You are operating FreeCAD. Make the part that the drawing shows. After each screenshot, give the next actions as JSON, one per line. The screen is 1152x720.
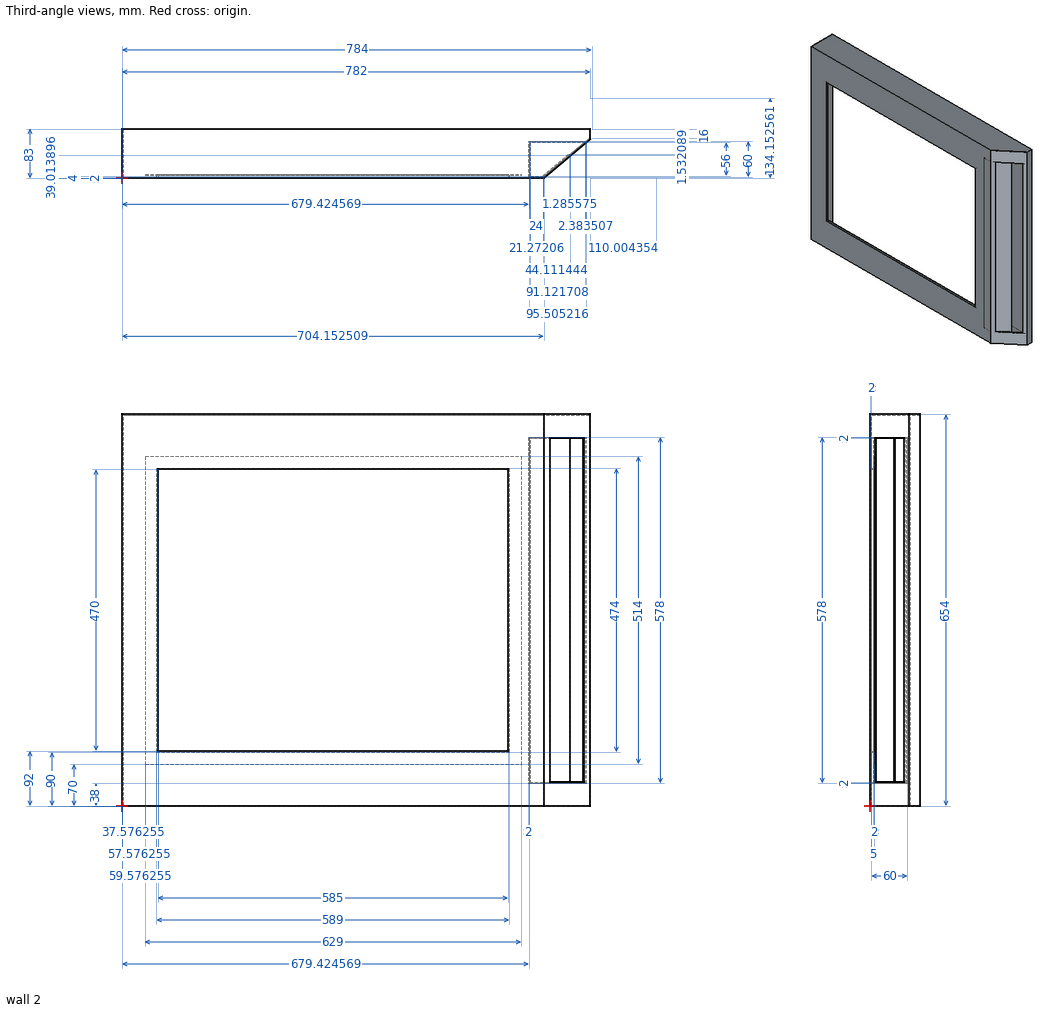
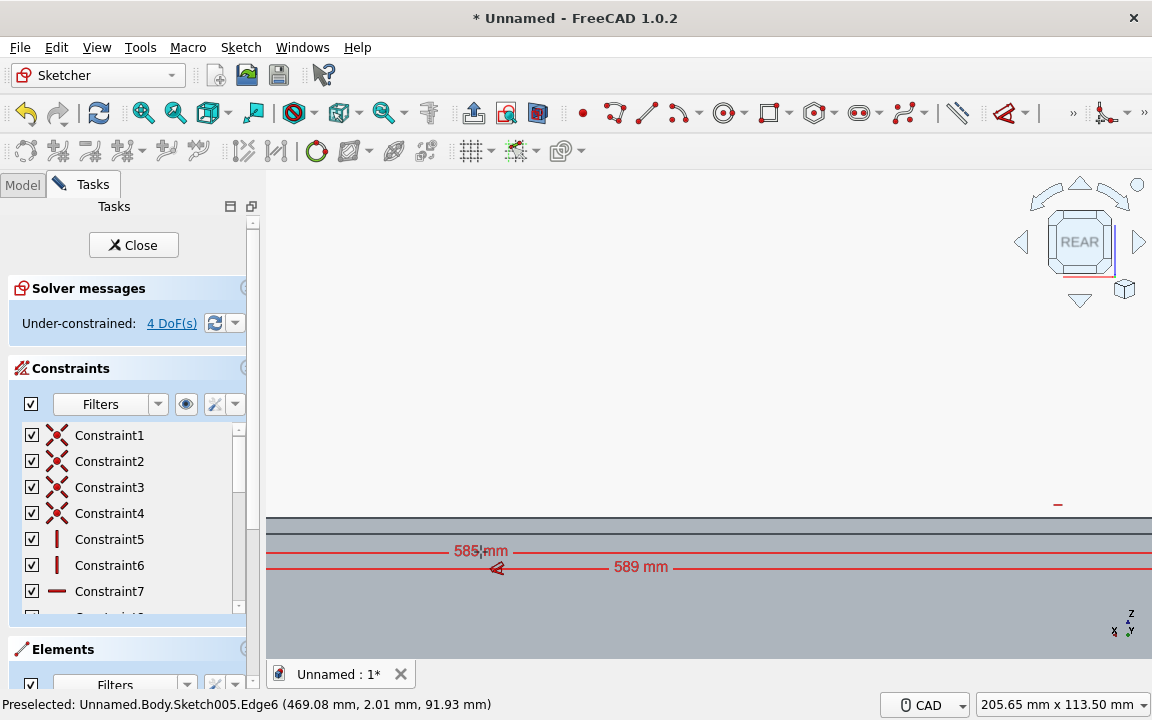
{"action": "scroll", "coordinate": [555, 526], "scroll_direction": "down", "scroll_amount": 10}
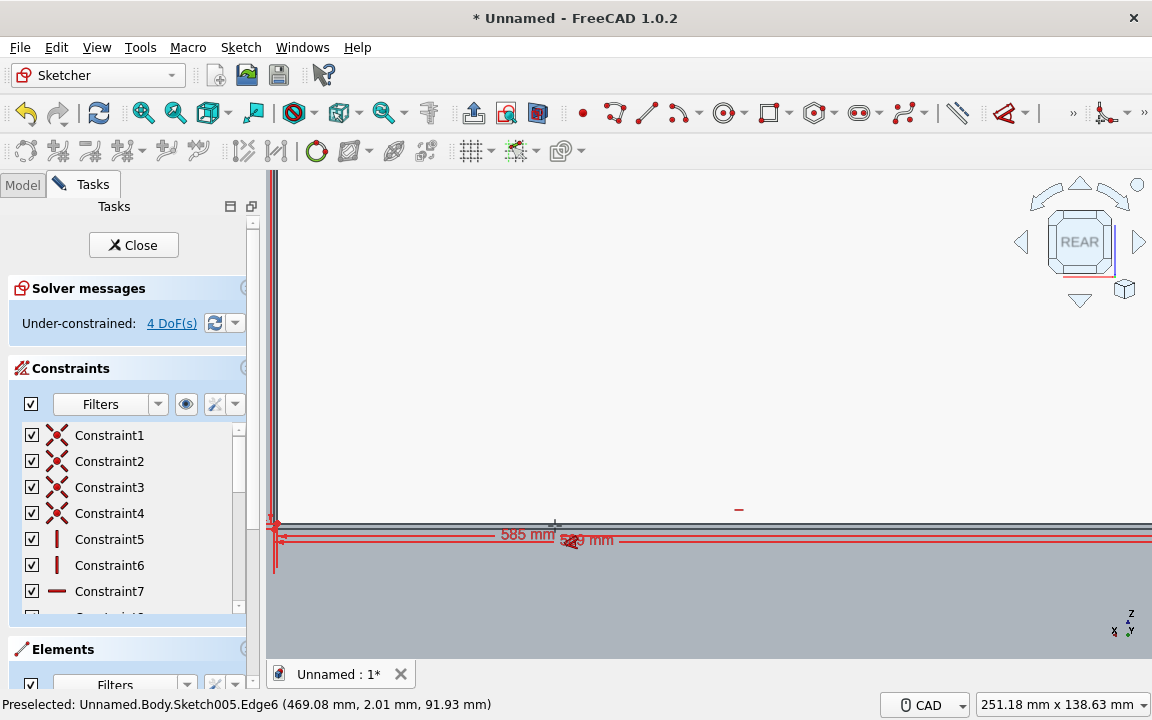
{"action": "scroll", "coordinate": [452, 528], "scroll_direction": "up", "scroll_amount": 9}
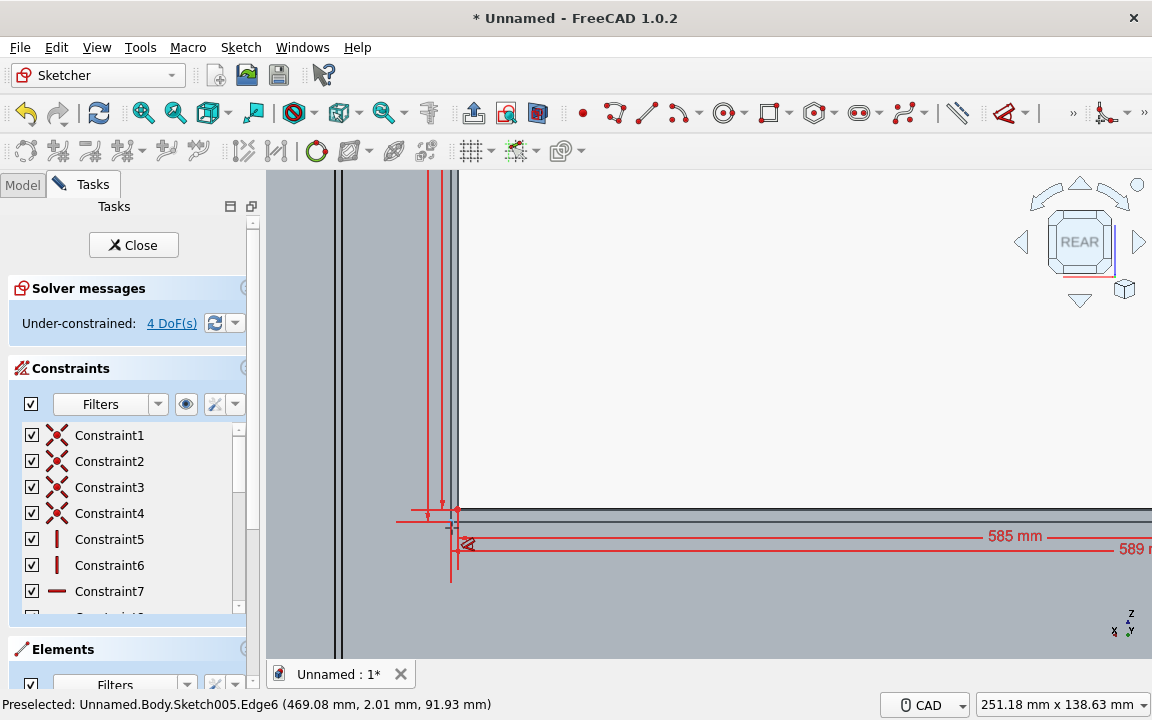
{"action": "left_click", "coordinate": [451, 522]}
{"action": "left_click", "coordinate": [417, 577]}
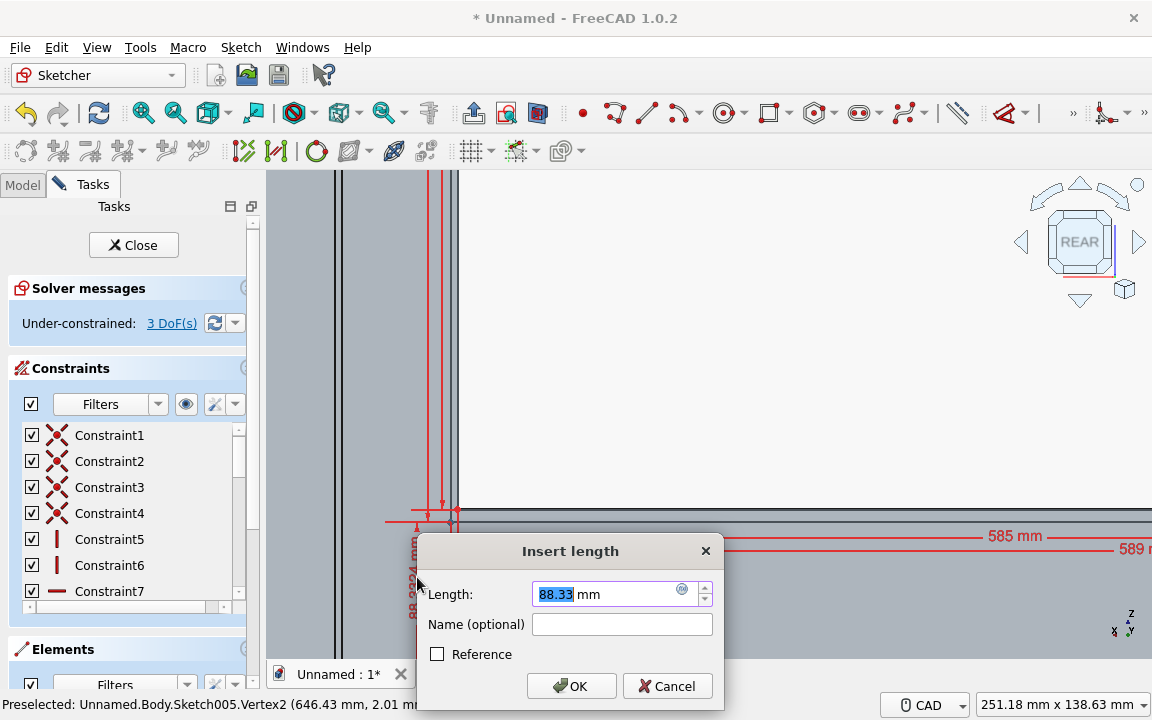
{"action": "type", "text": "90"}
{"action": "key", "text": "Return"}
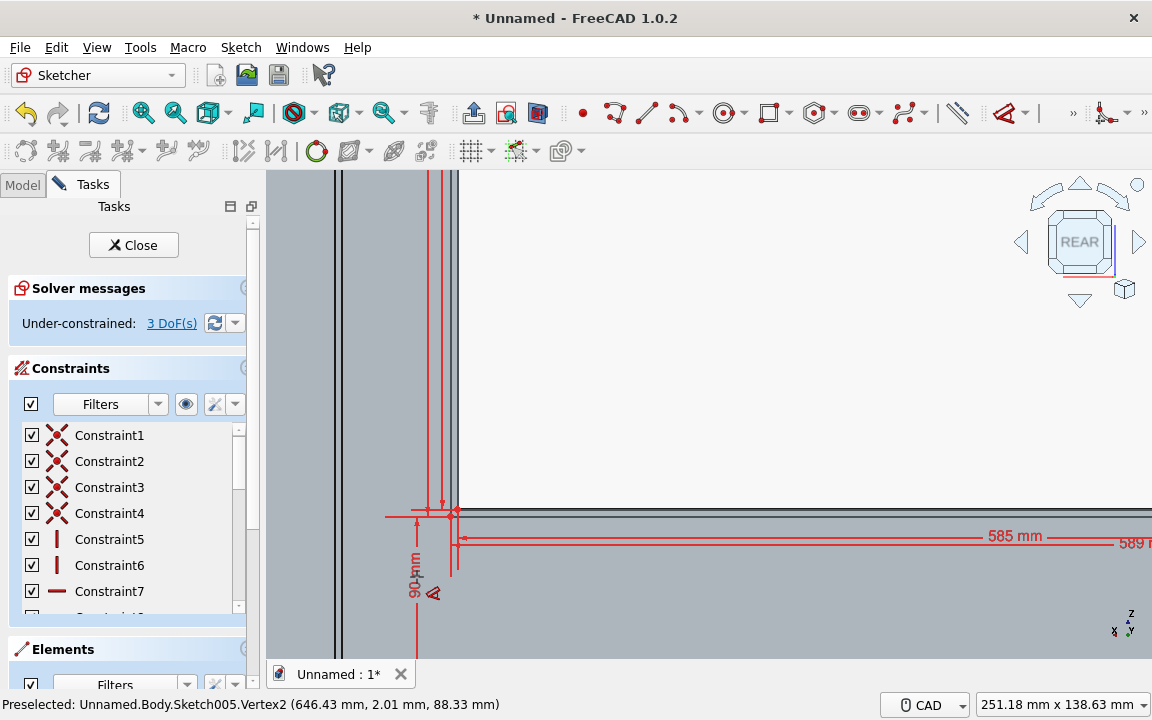
{"action": "scroll", "coordinate": [458, 510], "scroll_direction": "up", "scroll_amount": 2}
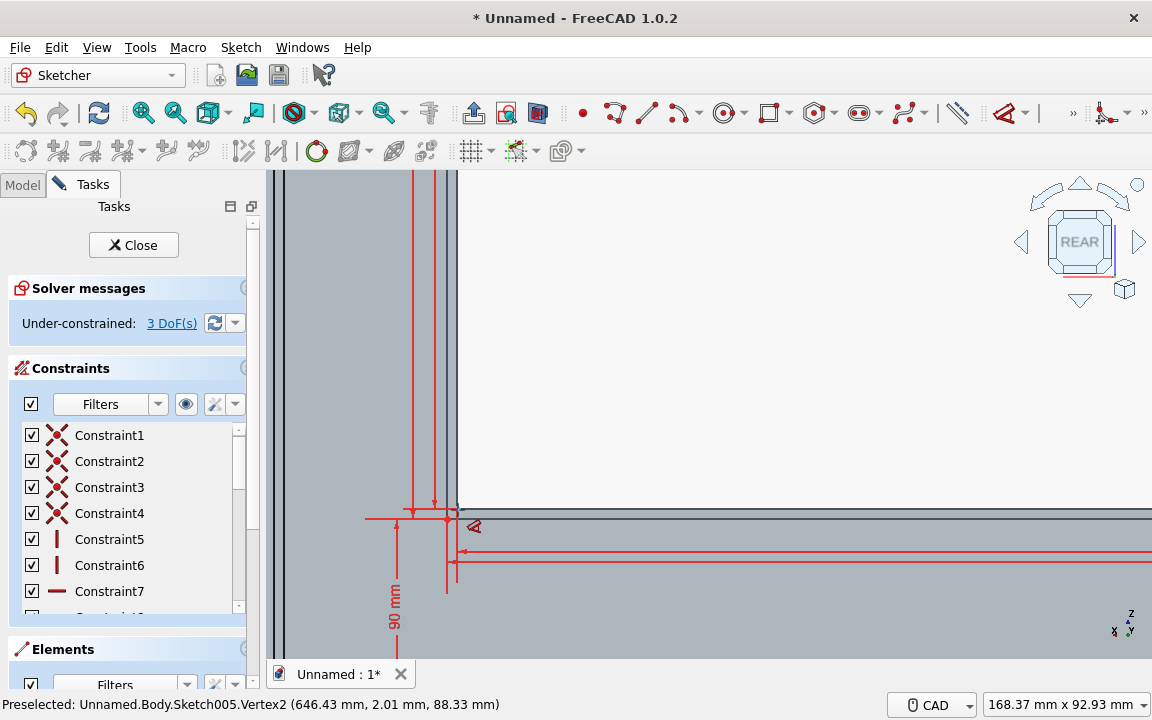
{"action": "left_click", "coordinate": [457, 509]}
{"action": "left_click", "coordinate": [423, 570]}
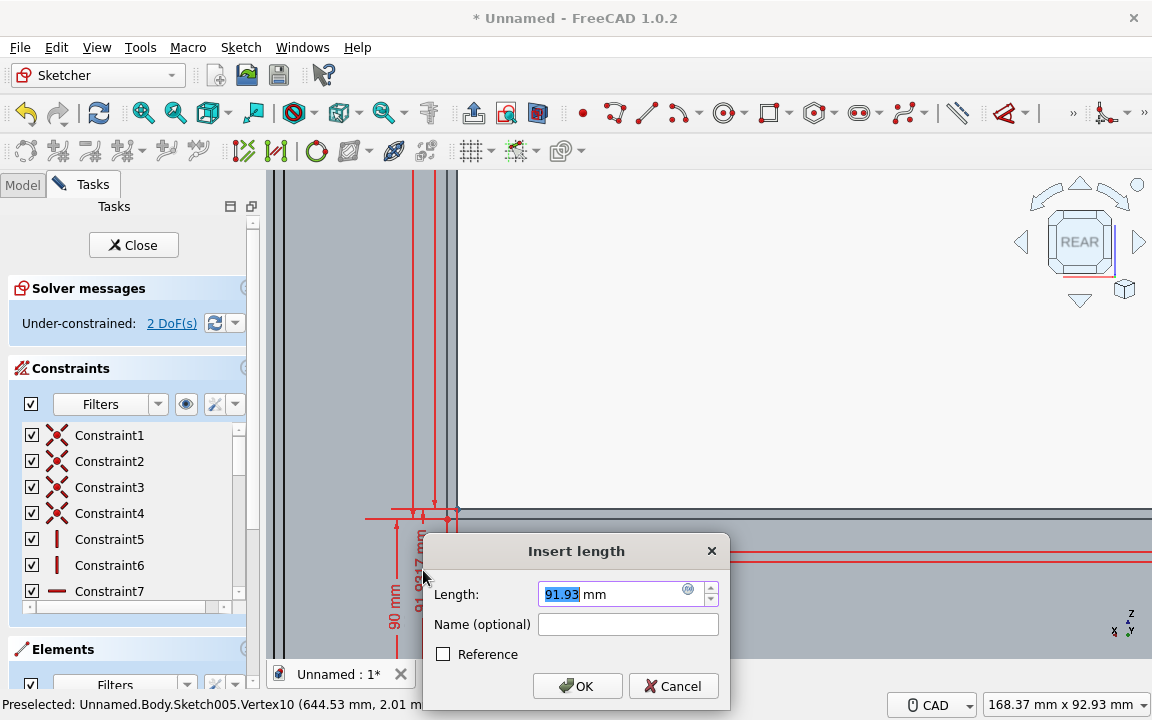
{"action": "type", "text": "92"}
{"action": "key", "text": "Return"}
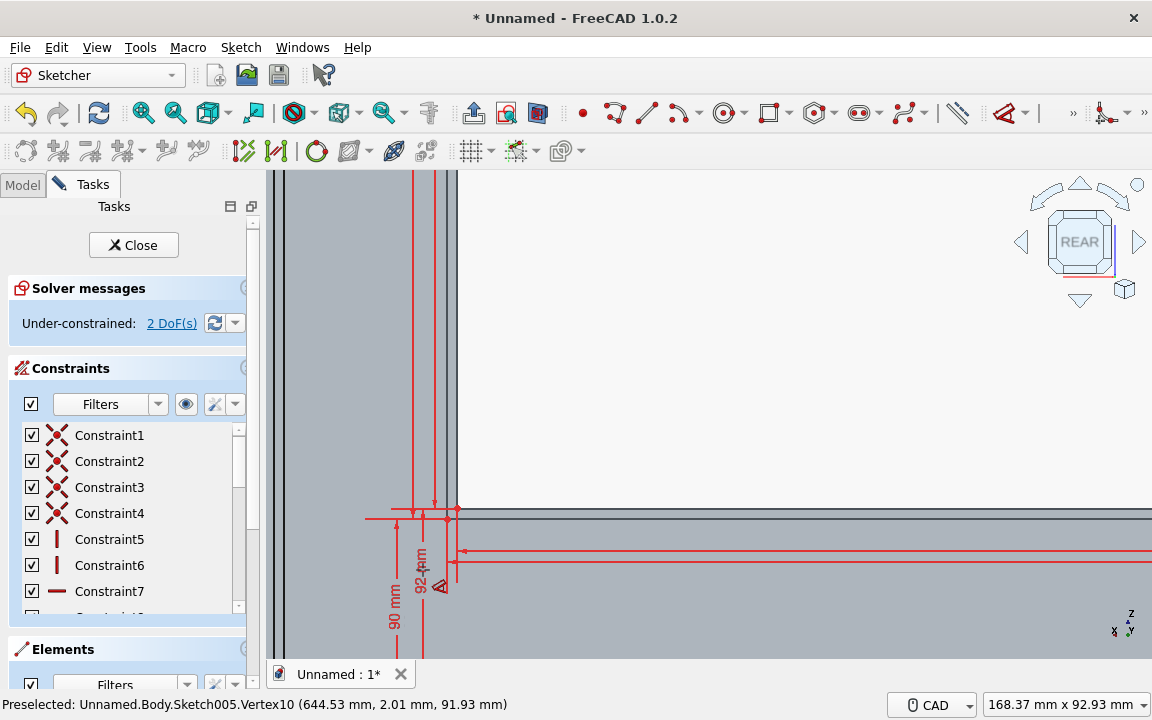
{"action": "scroll", "coordinate": [453, 527], "scroll_direction": "down", "scroll_amount": 11}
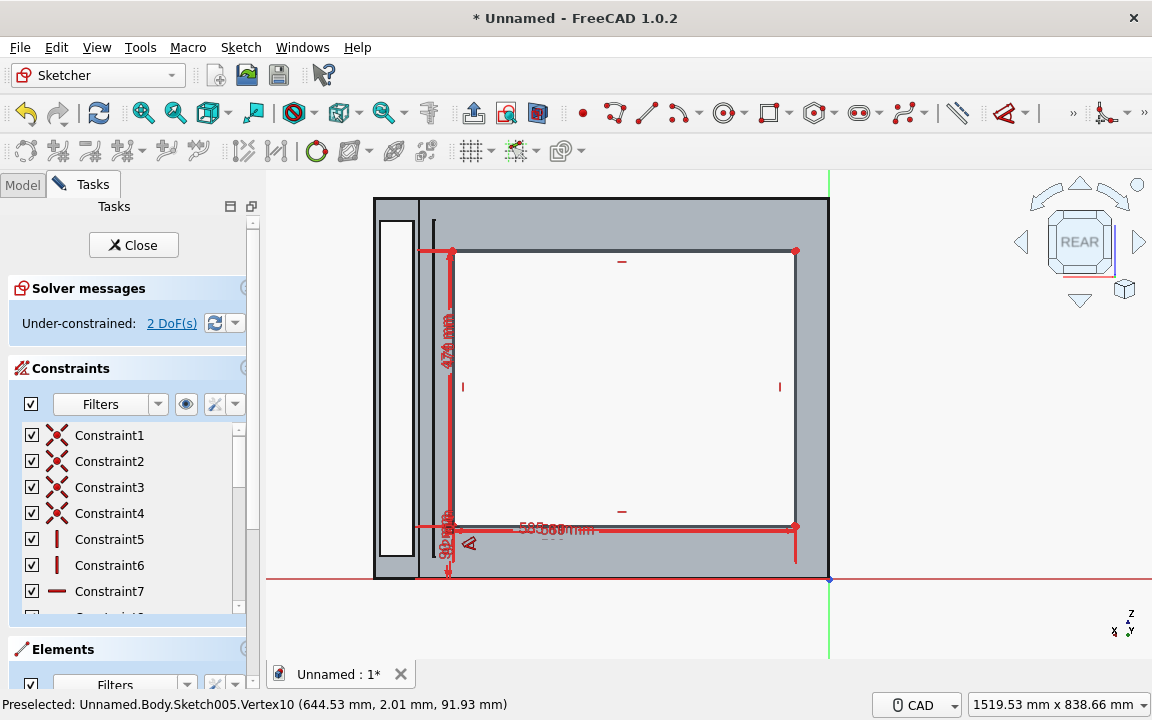
{"action": "scroll", "coordinate": [796, 527], "scroll_direction": "up", "scroll_amount": 10}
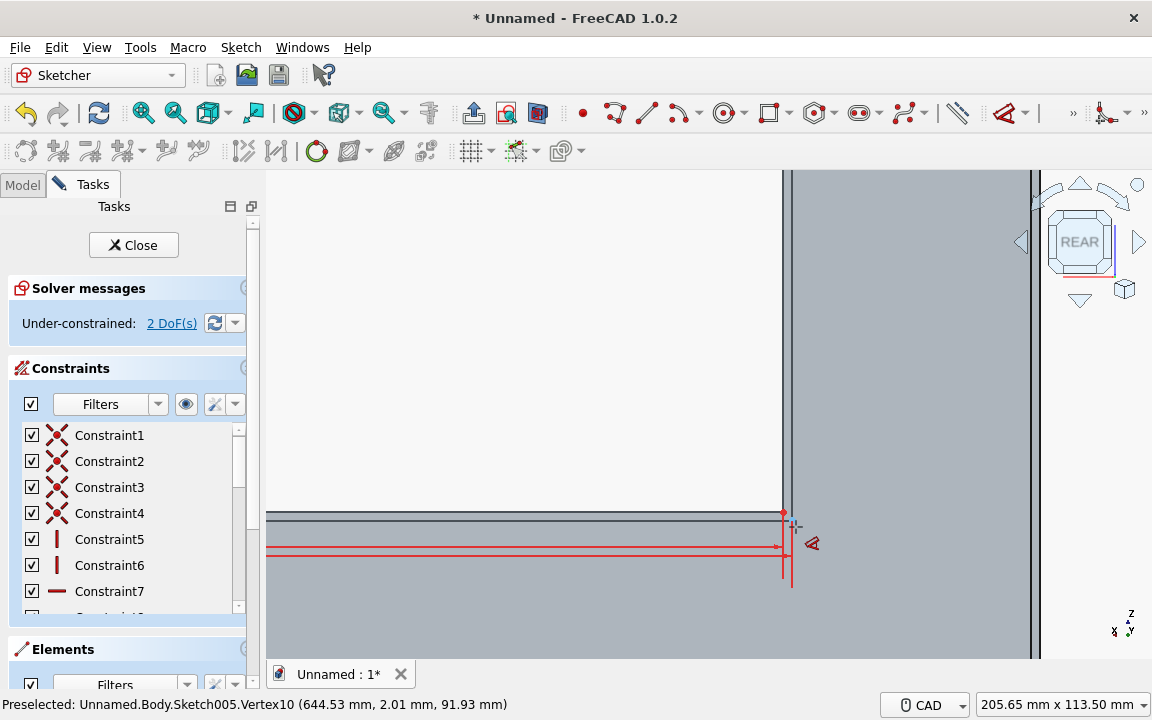
{"action": "left_click", "coordinate": [792, 521]}
{"action": "left_click", "coordinate": [890, 487]}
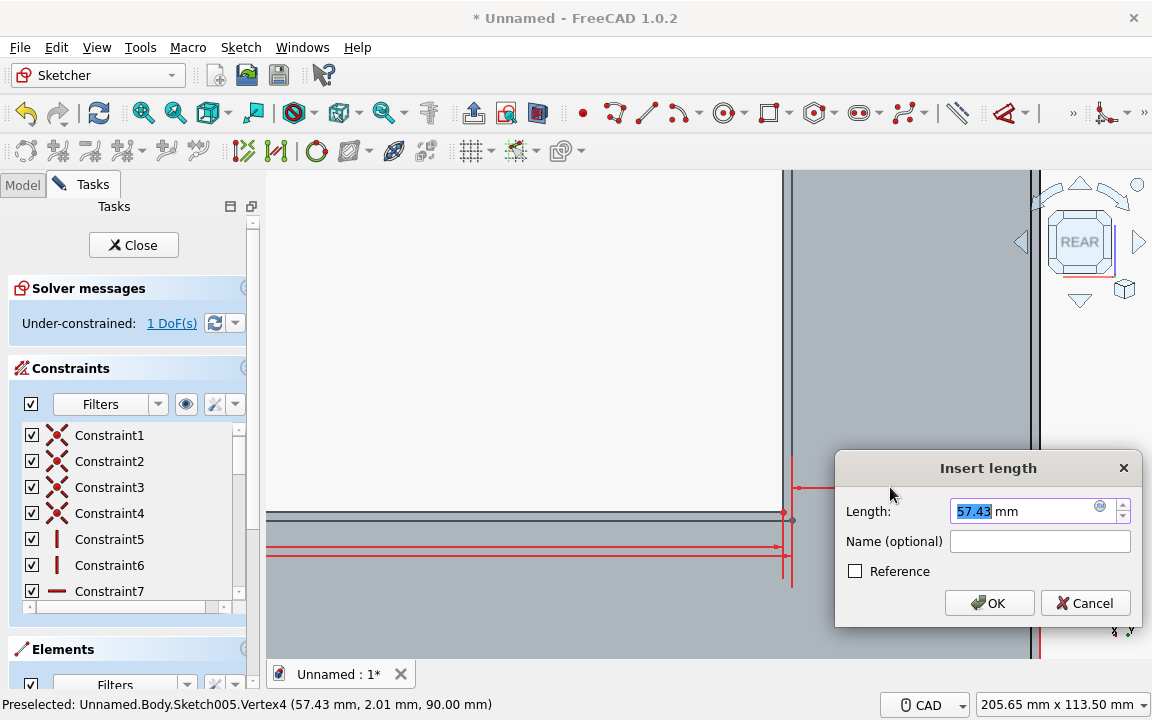
{"action": "type", "text": "57.576255"}
{"action": "key", "text": "Return"}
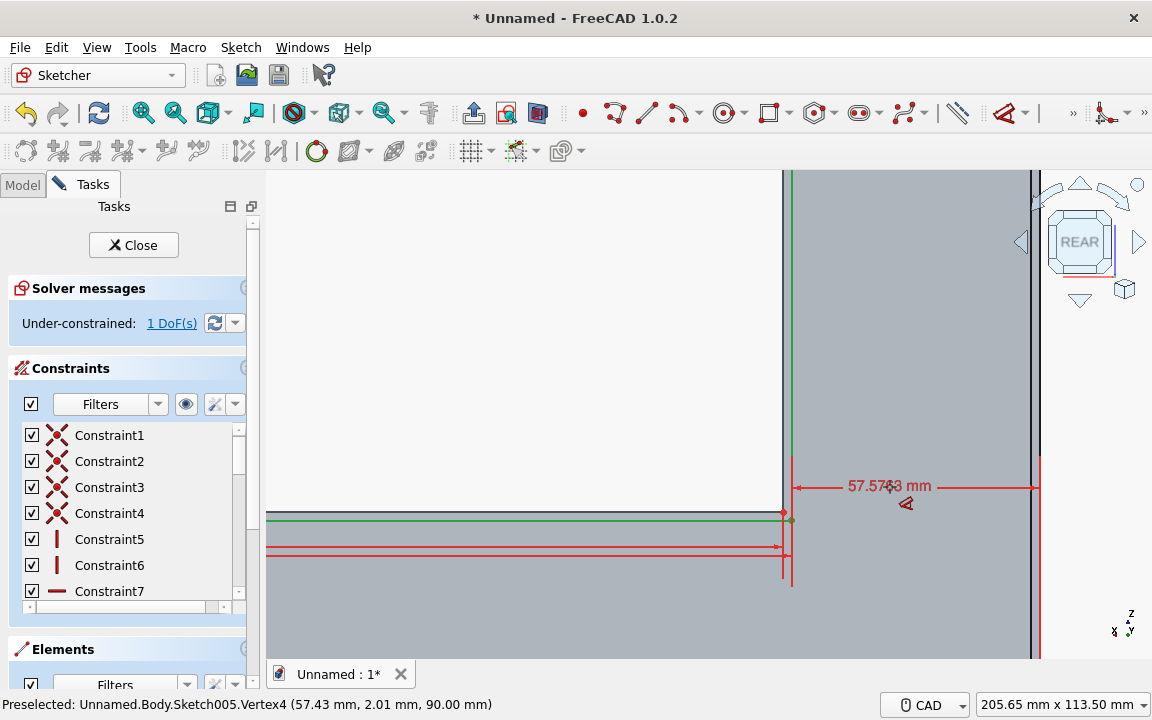
{"action": "left_click", "coordinate": [783, 512]}
{"action": "left_click", "coordinate": [814, 478]}